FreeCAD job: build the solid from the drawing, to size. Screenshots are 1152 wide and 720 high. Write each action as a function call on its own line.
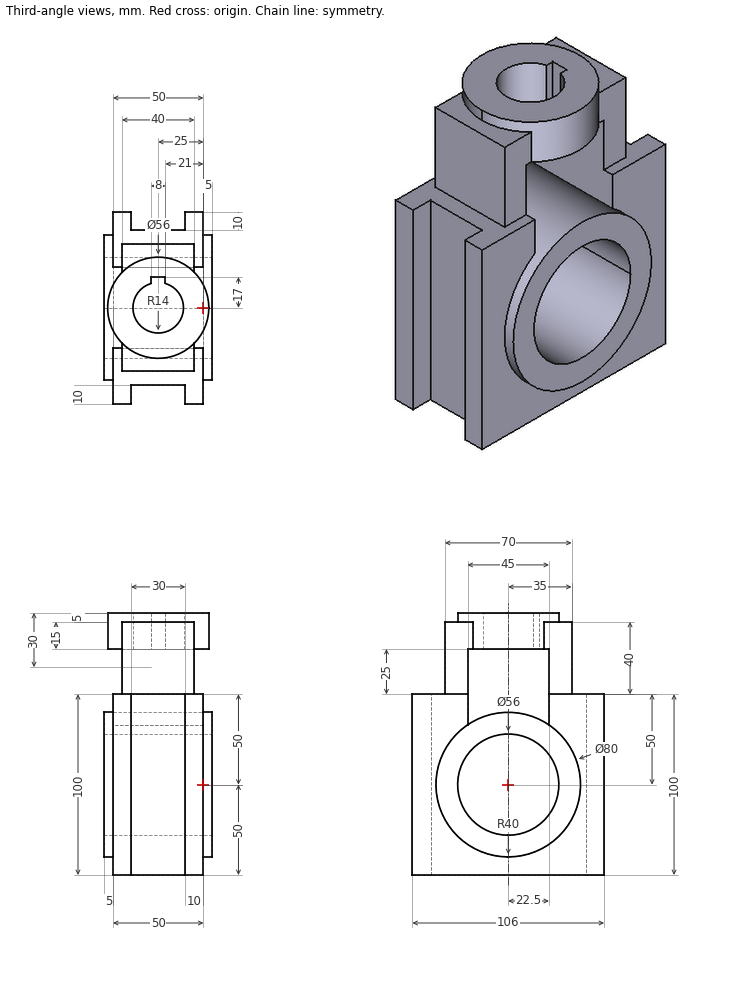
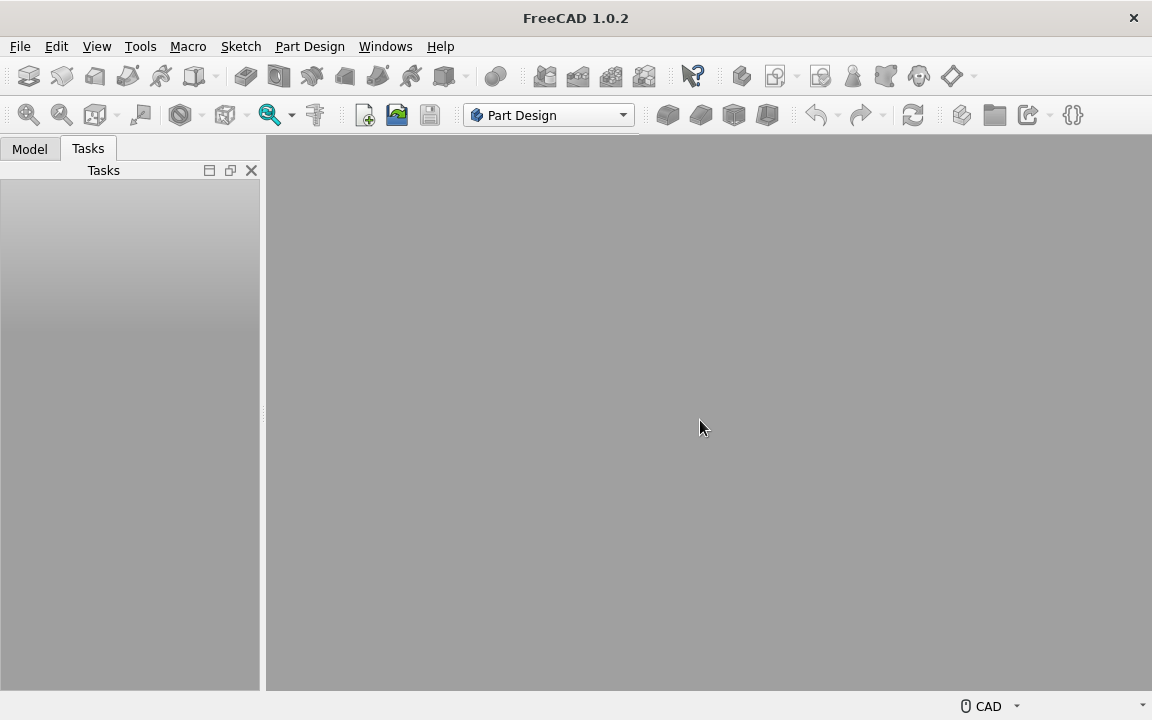
key(ctrl+n)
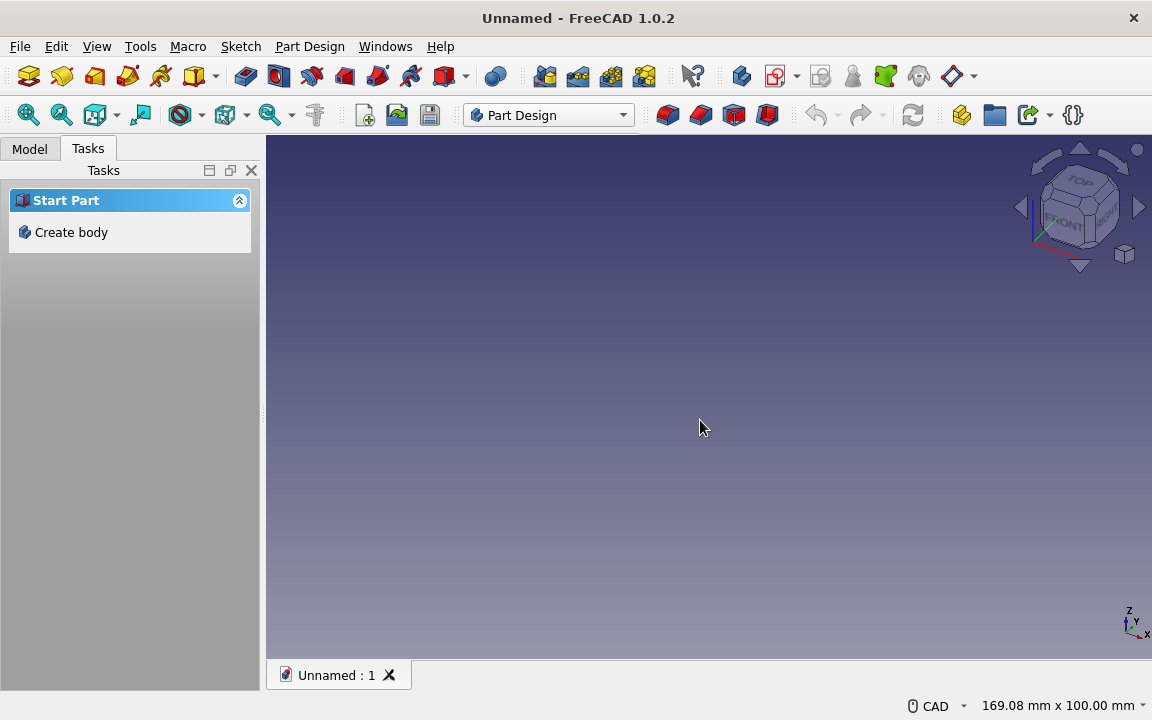
click(774, 76)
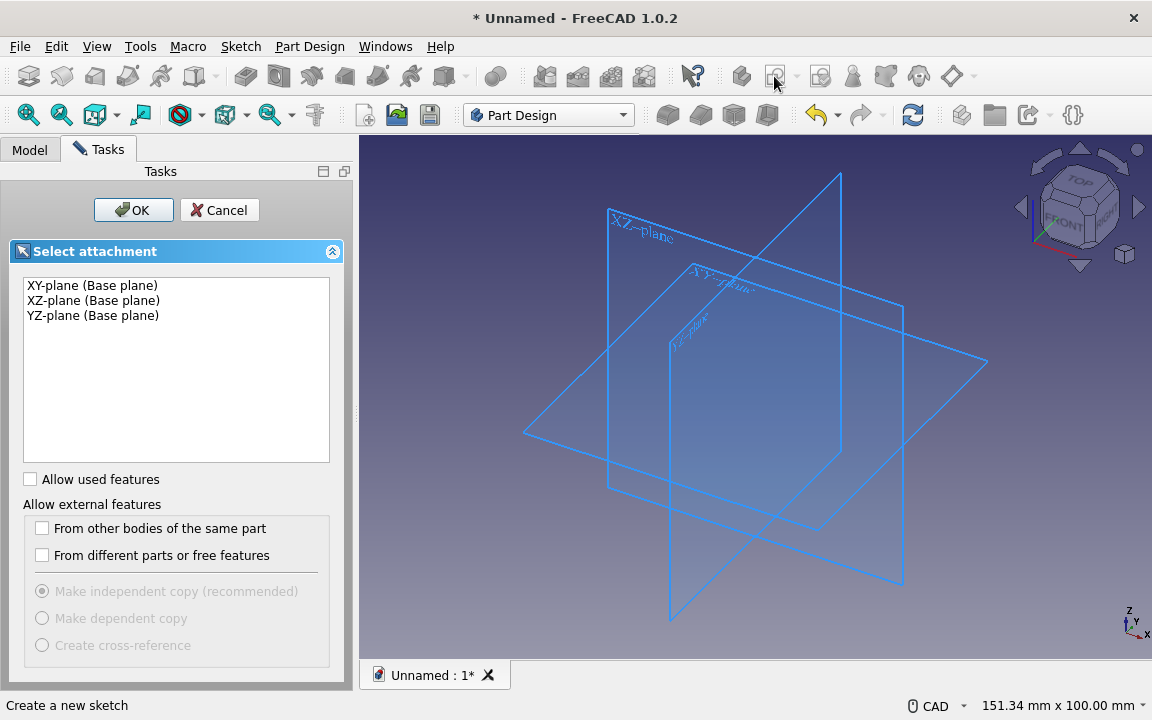
click(84, 316)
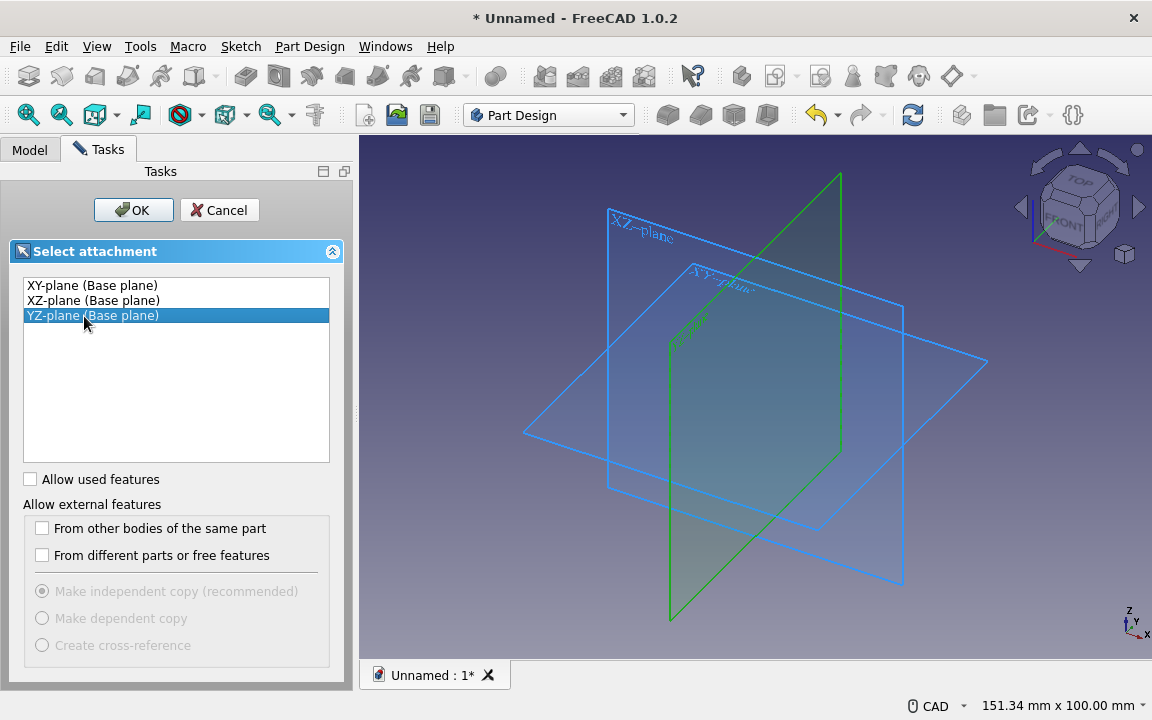
click(134, 210)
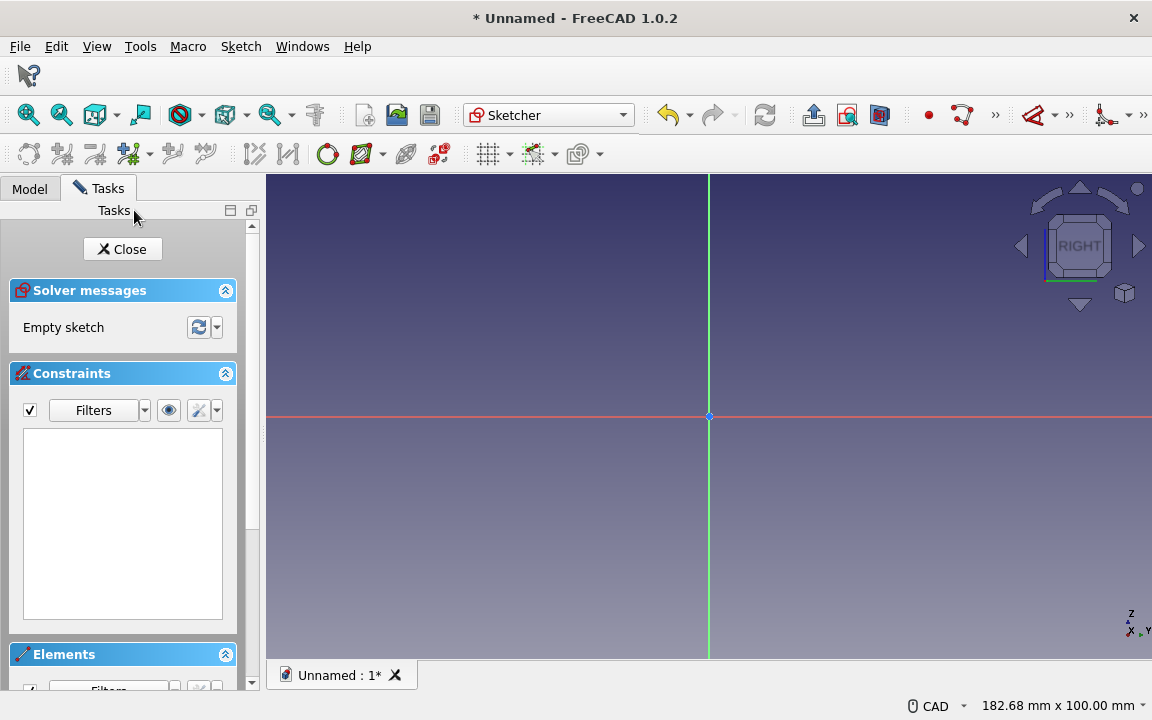
scroll(501, 416, down, 2)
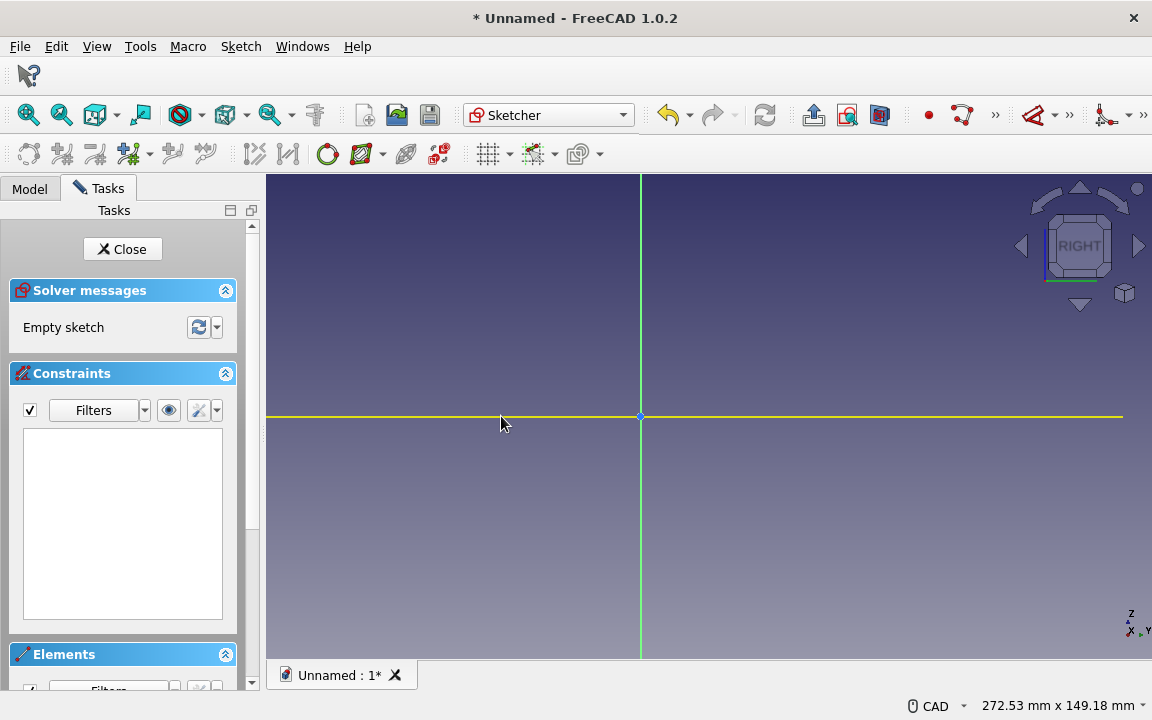
key(g)
key(v)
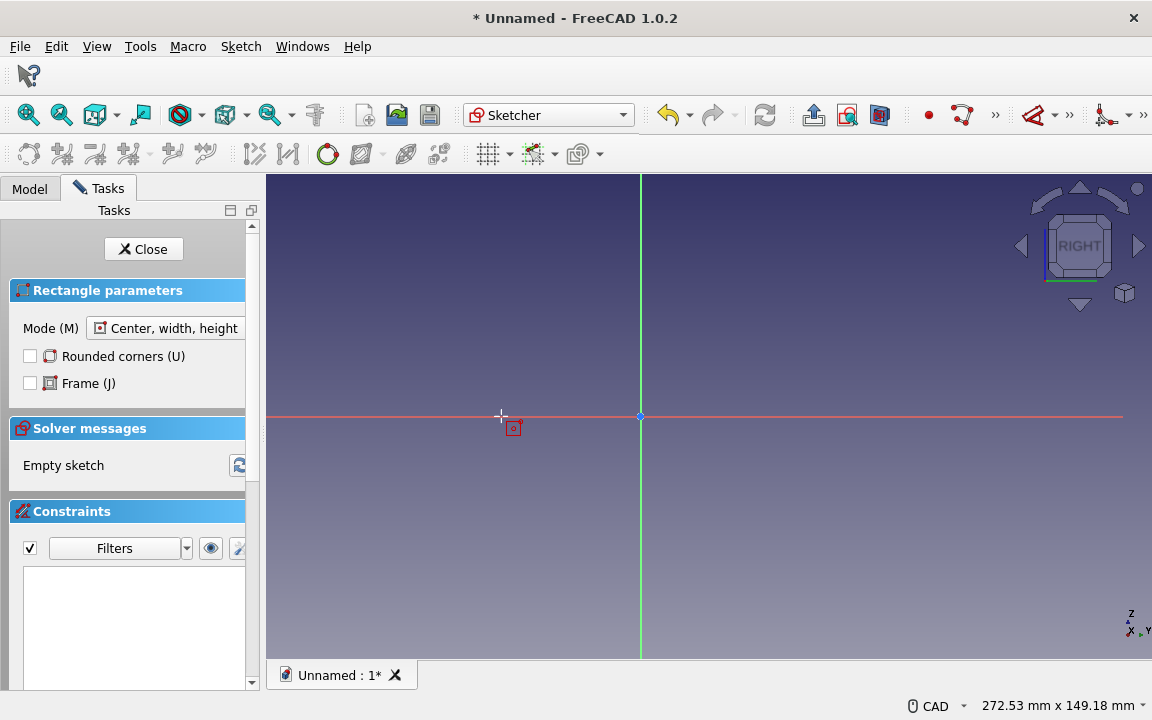
click(641, 416)
move(813, 254)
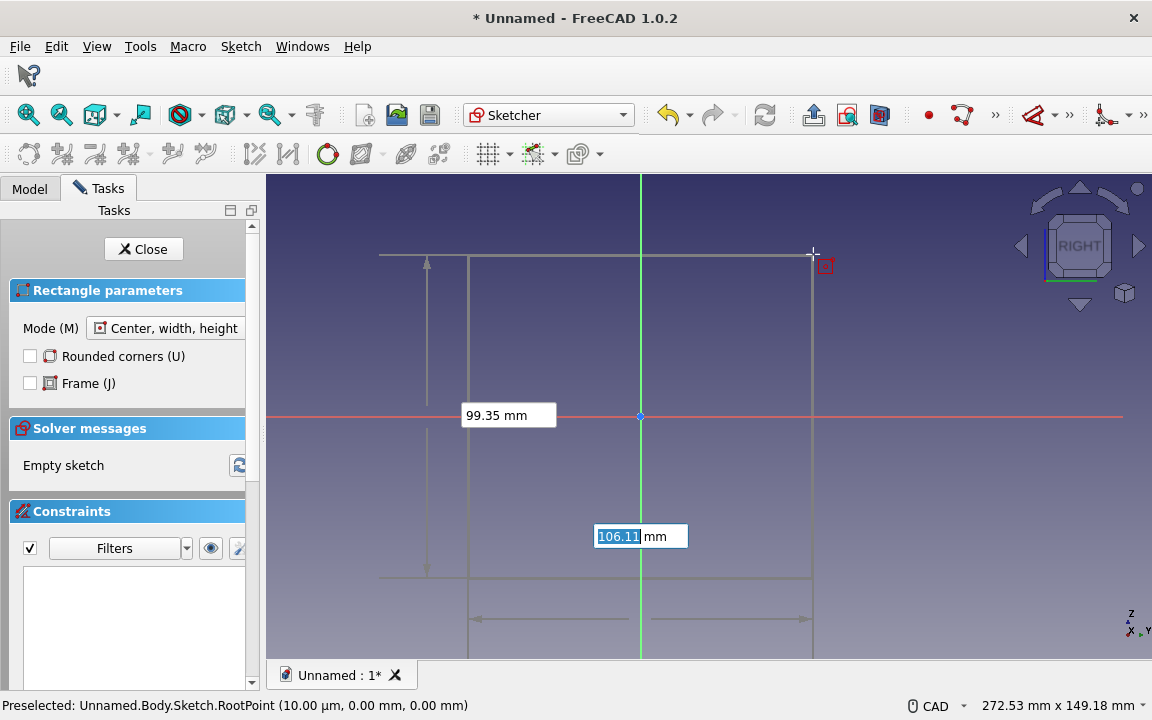
text(106)
key(Tab)
text(100)
key(Return)
key(Escape)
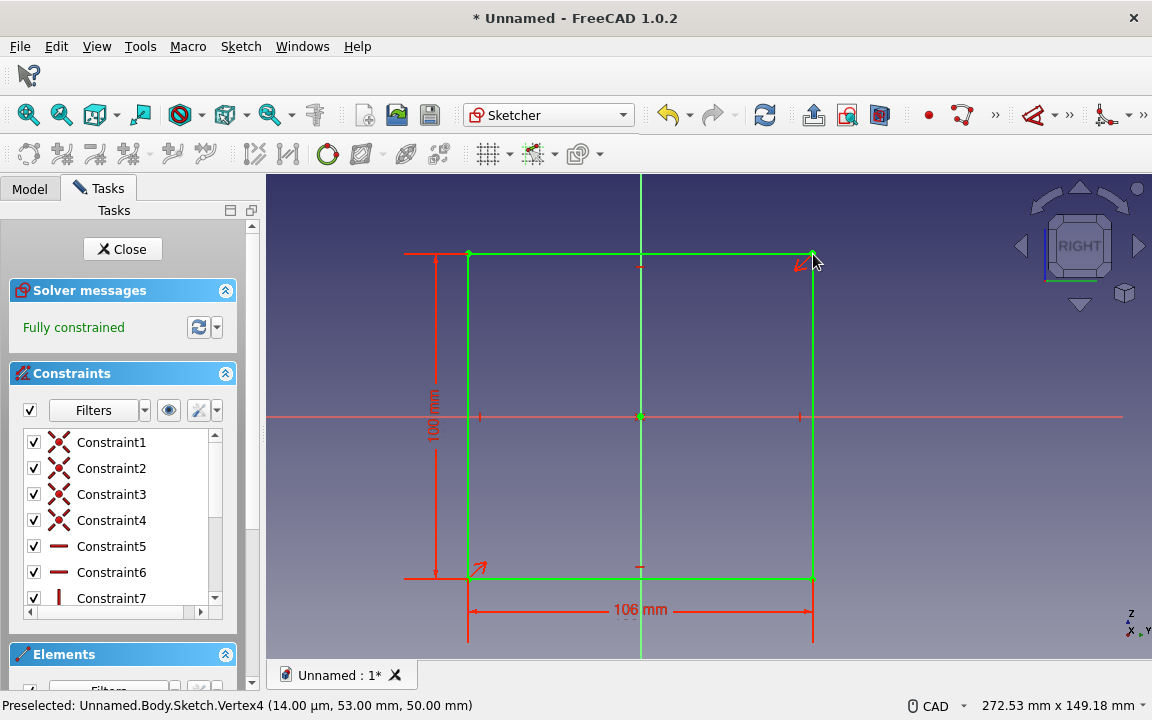
click(123, 249)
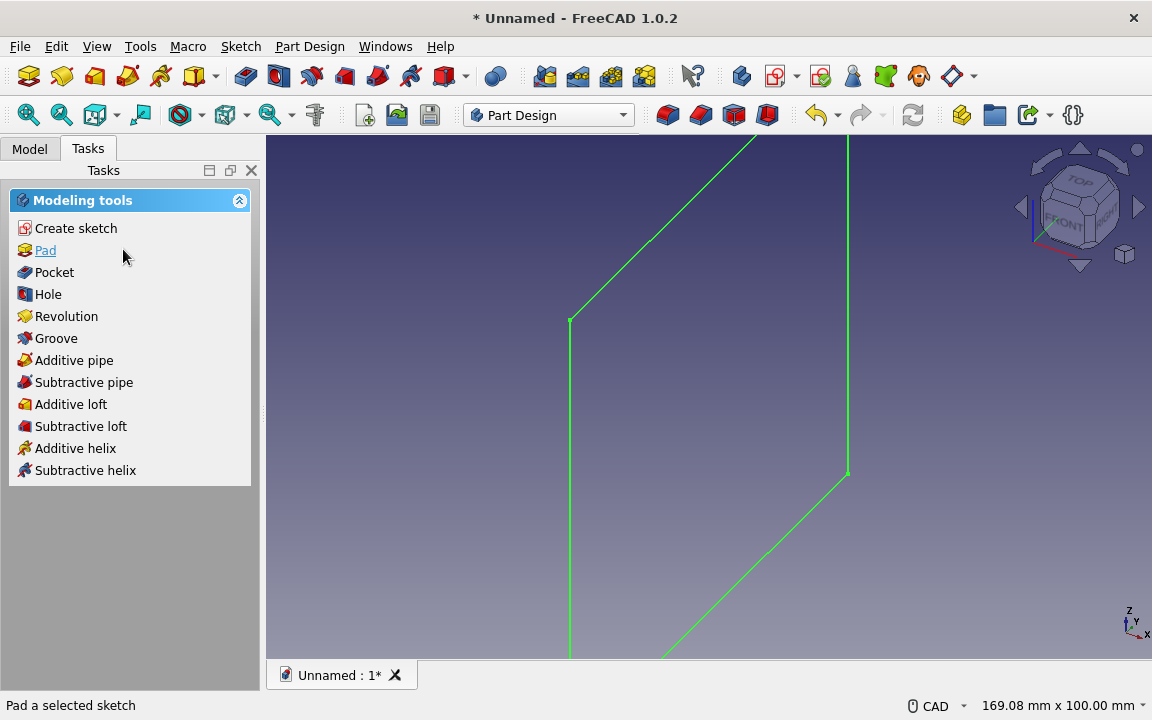
click(29, 76)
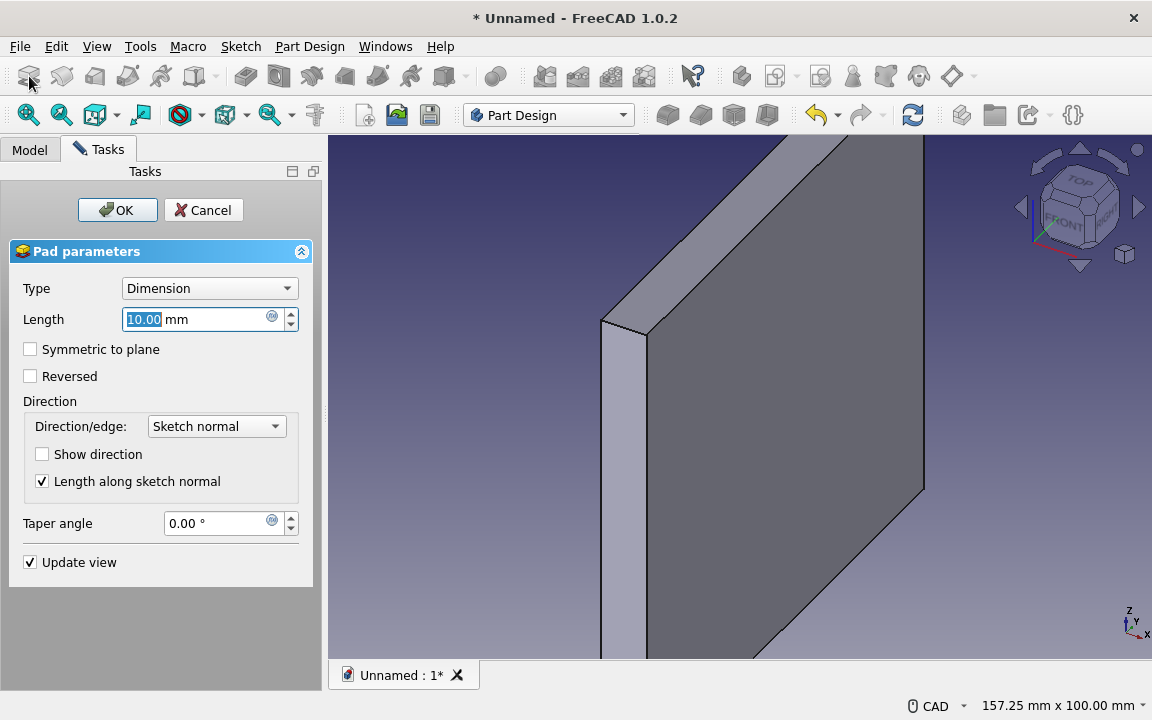
text(50)
key(Tab)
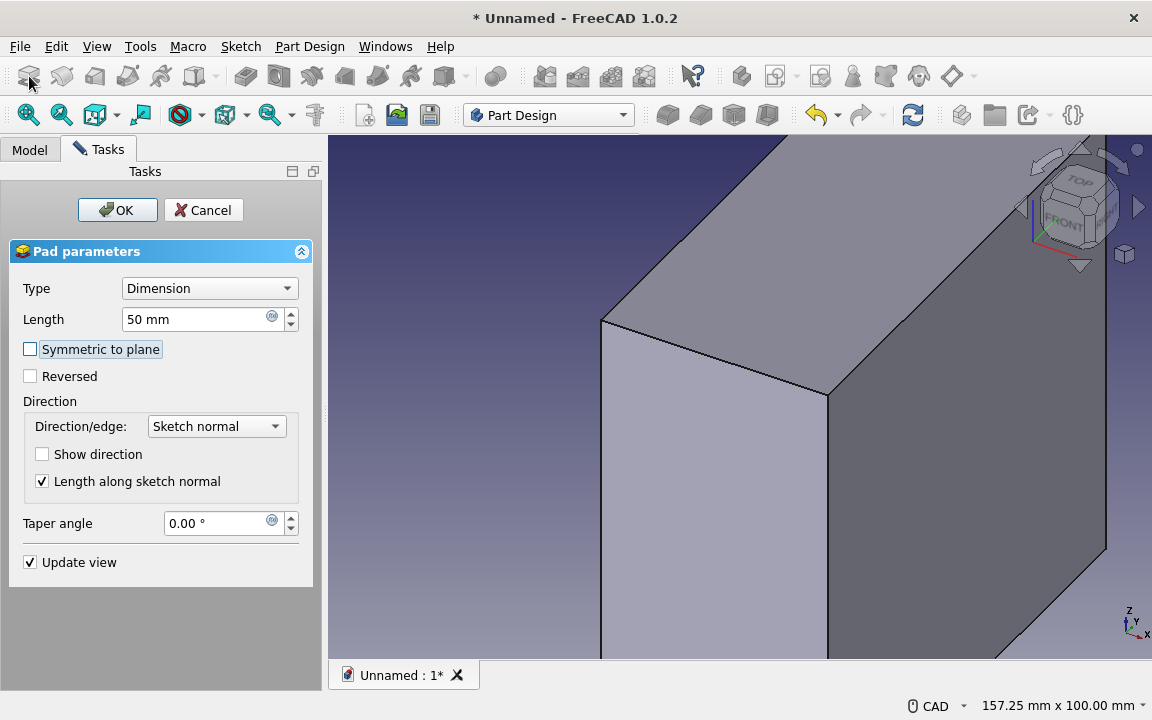
click(31, 376)